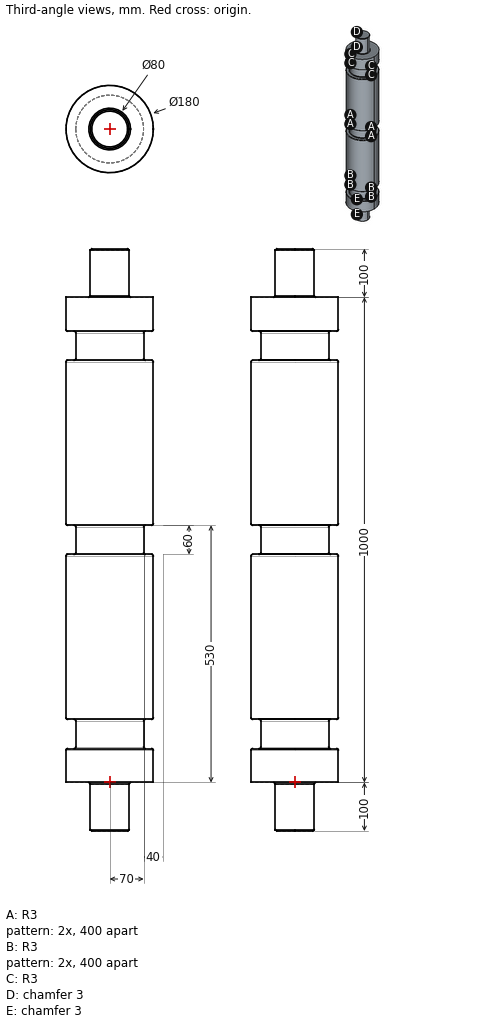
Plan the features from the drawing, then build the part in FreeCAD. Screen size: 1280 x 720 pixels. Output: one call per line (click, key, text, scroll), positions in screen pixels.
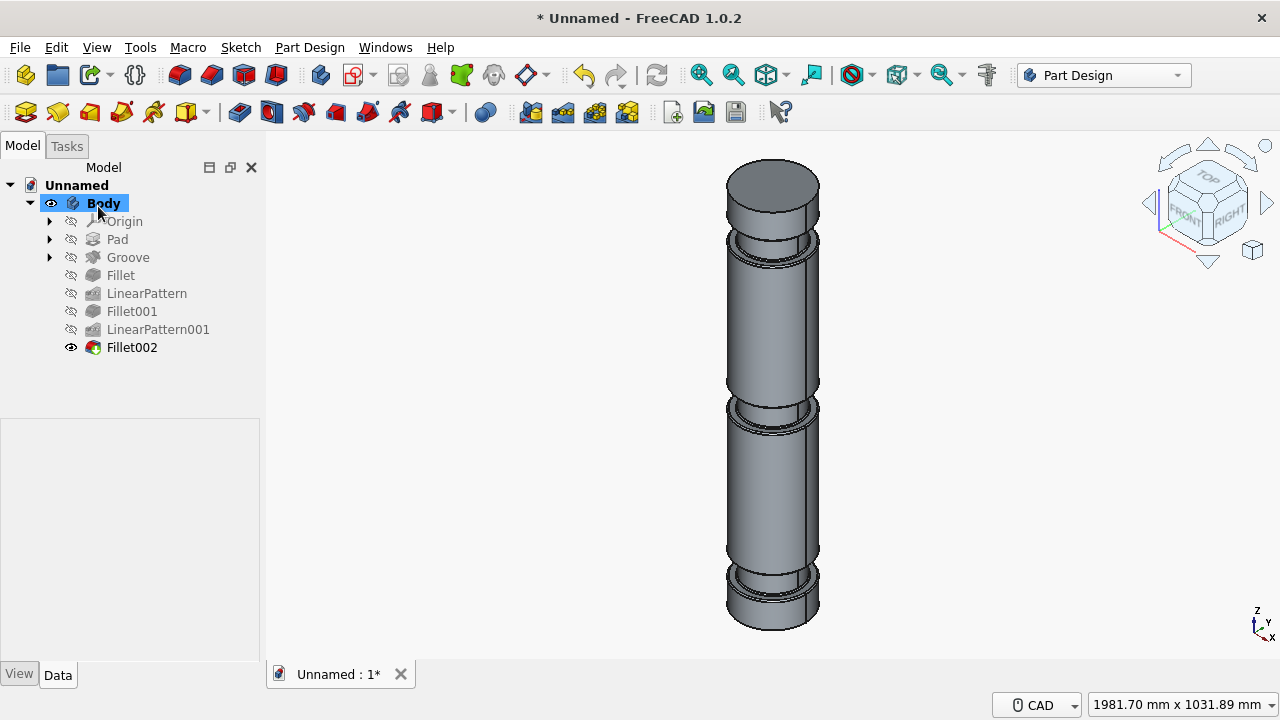
click(773, 185)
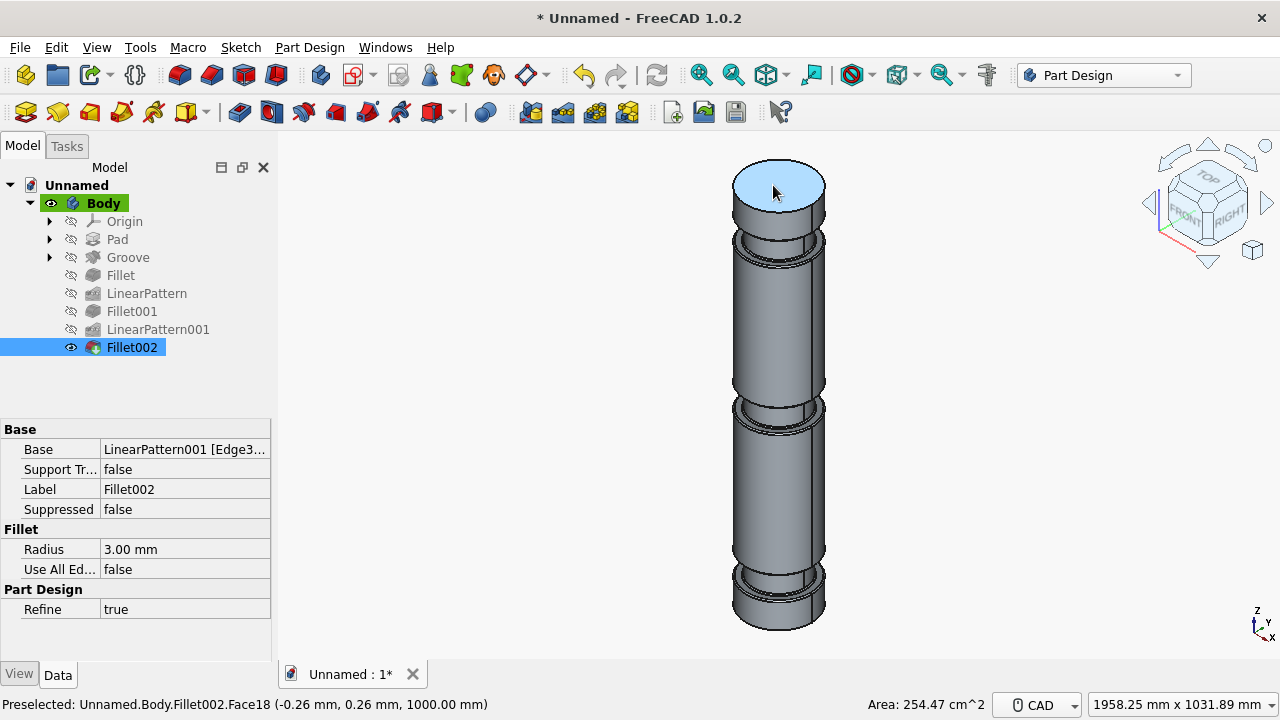
click(354, 76)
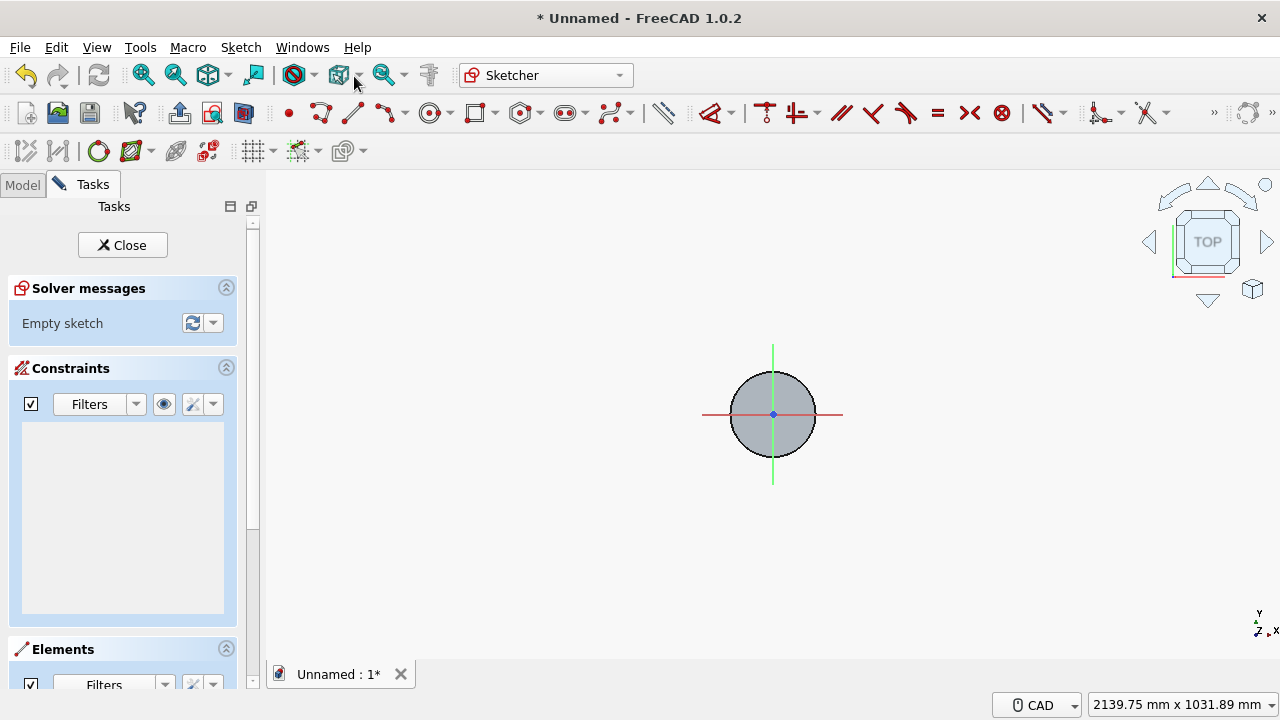
scroll(784, 415, up, 10)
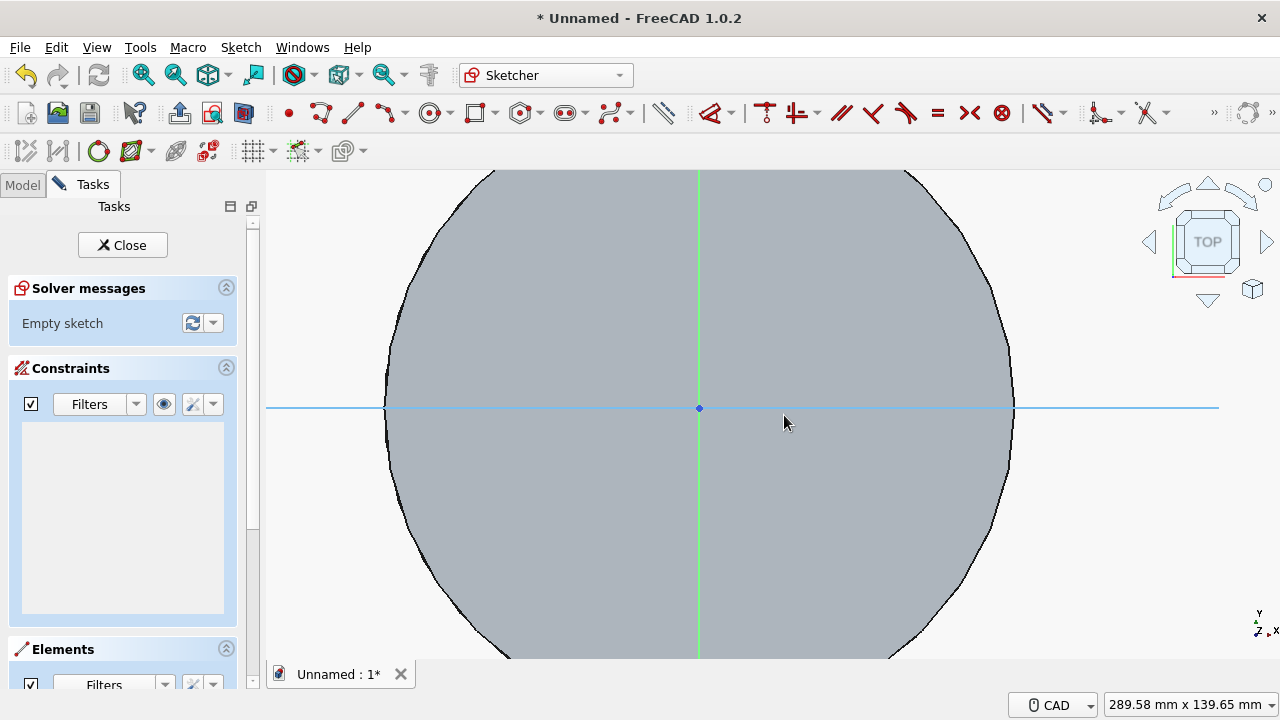
click(430, 114)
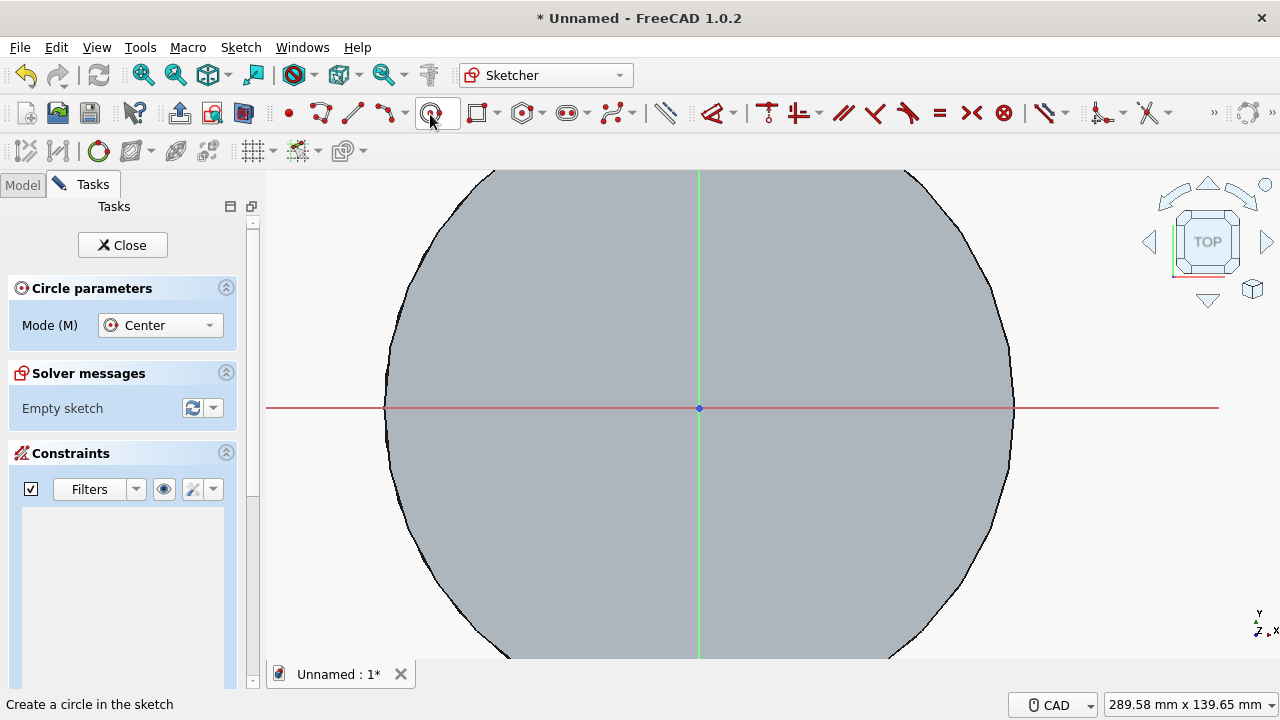
click(699, 408)
move(798, 309)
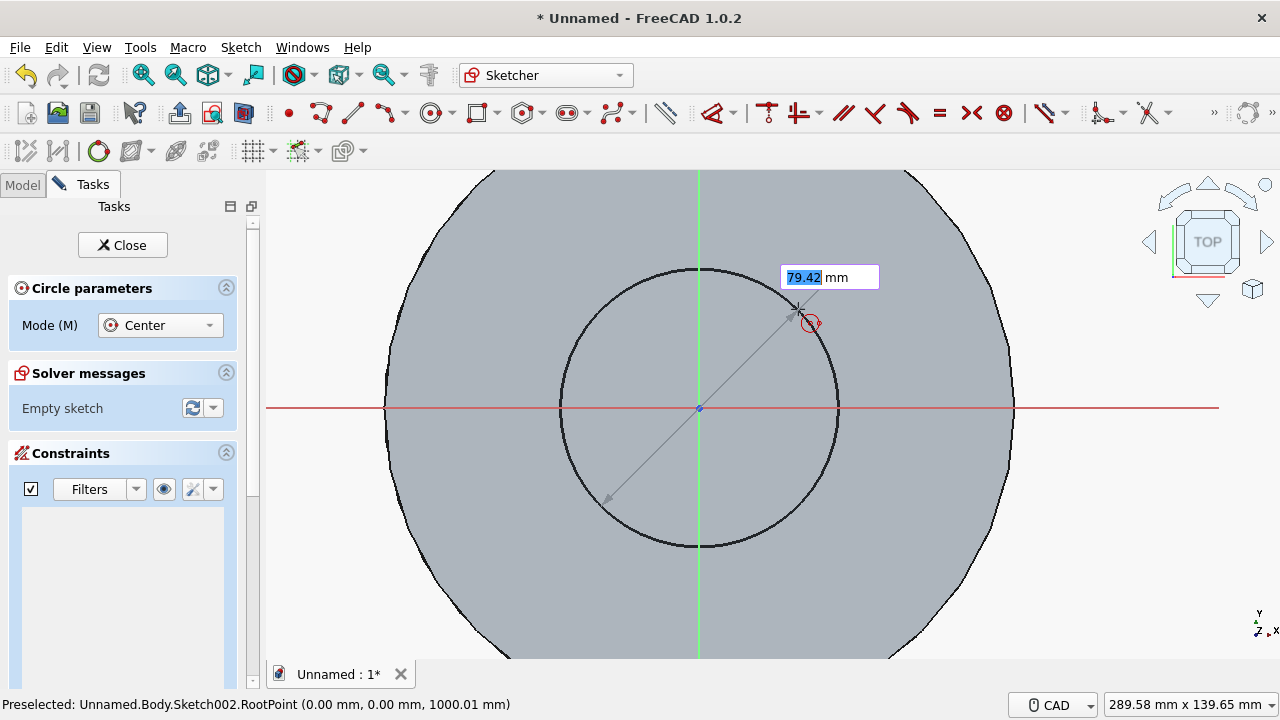
text(80)
key(Return)
key(Escape)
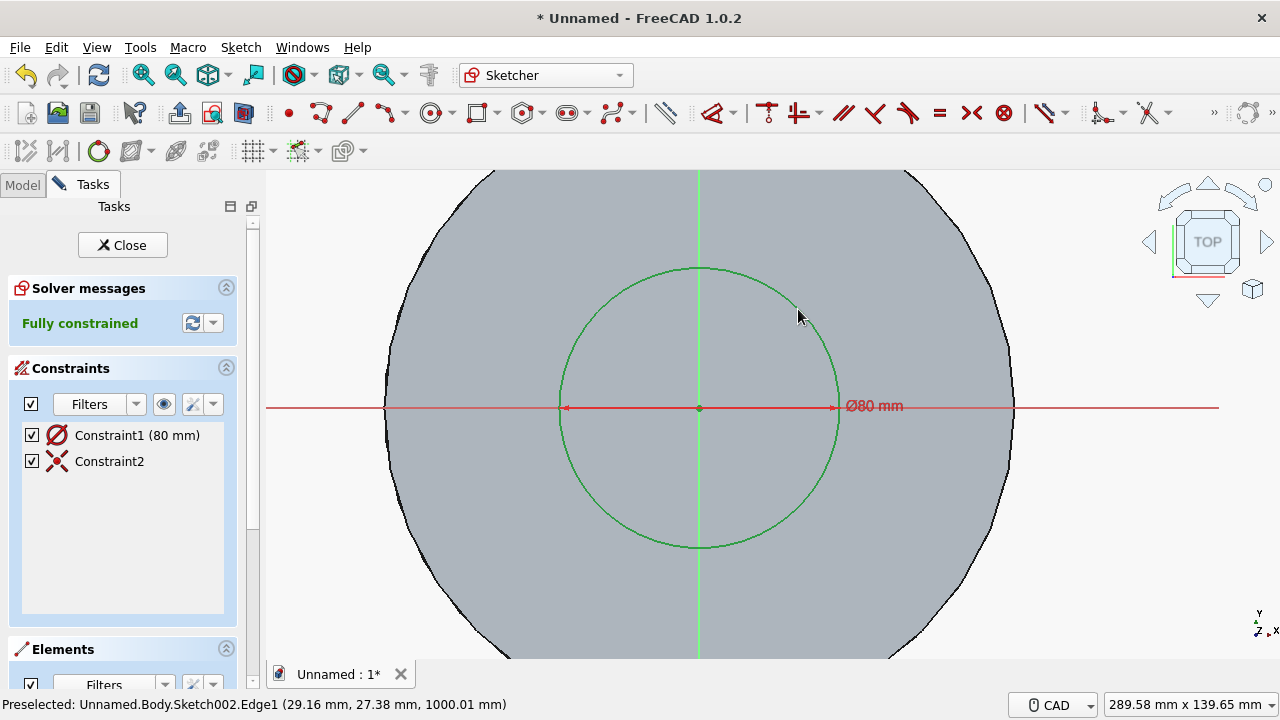
click(123, 245)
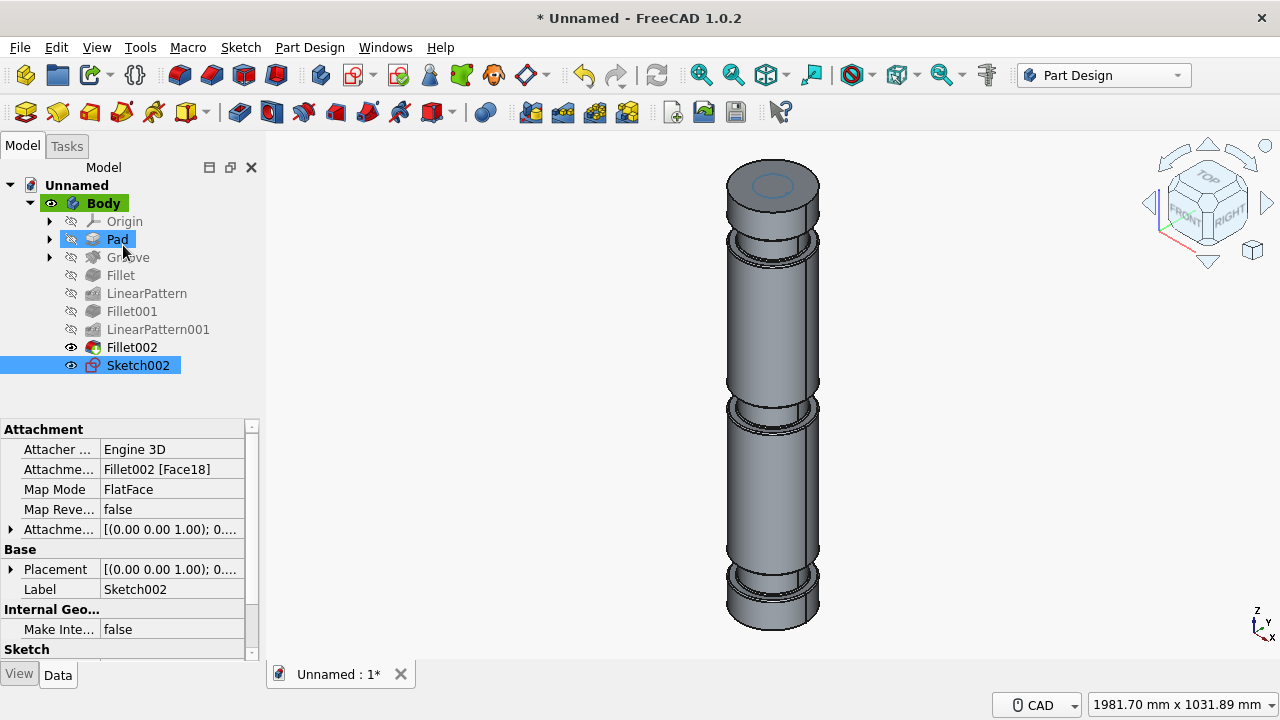
click(26, 112)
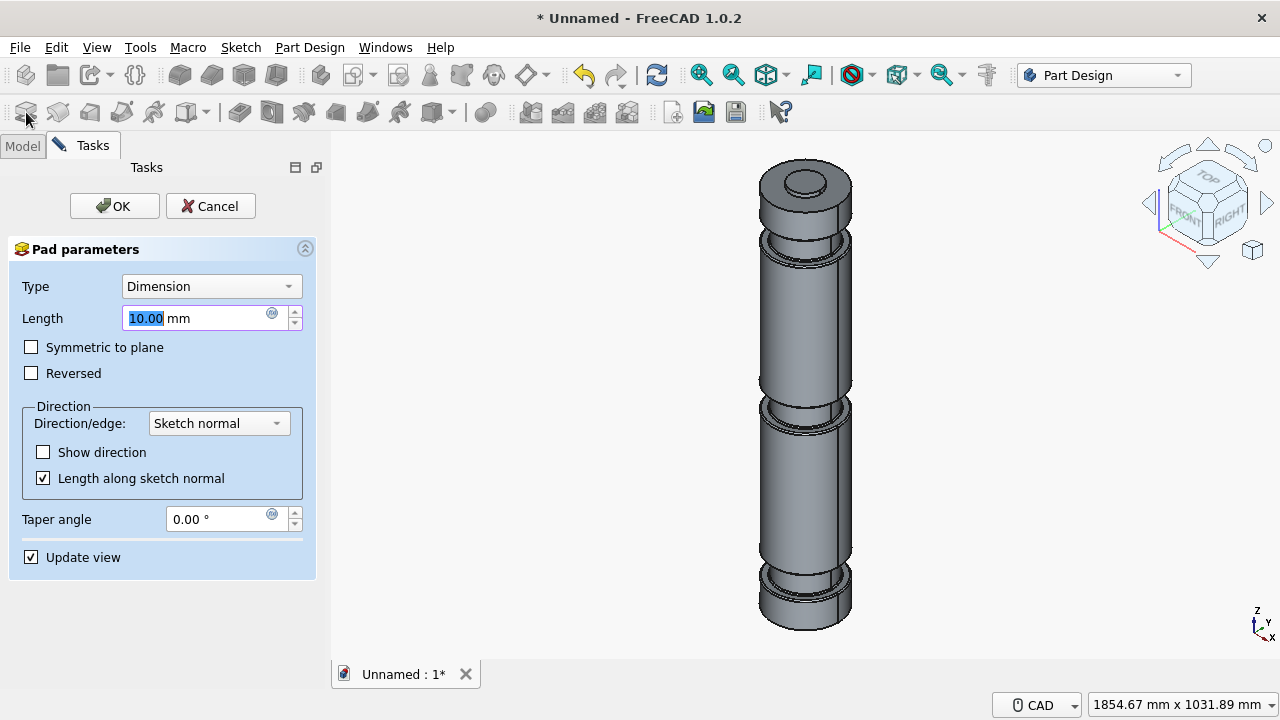
text(100)
key(Tab)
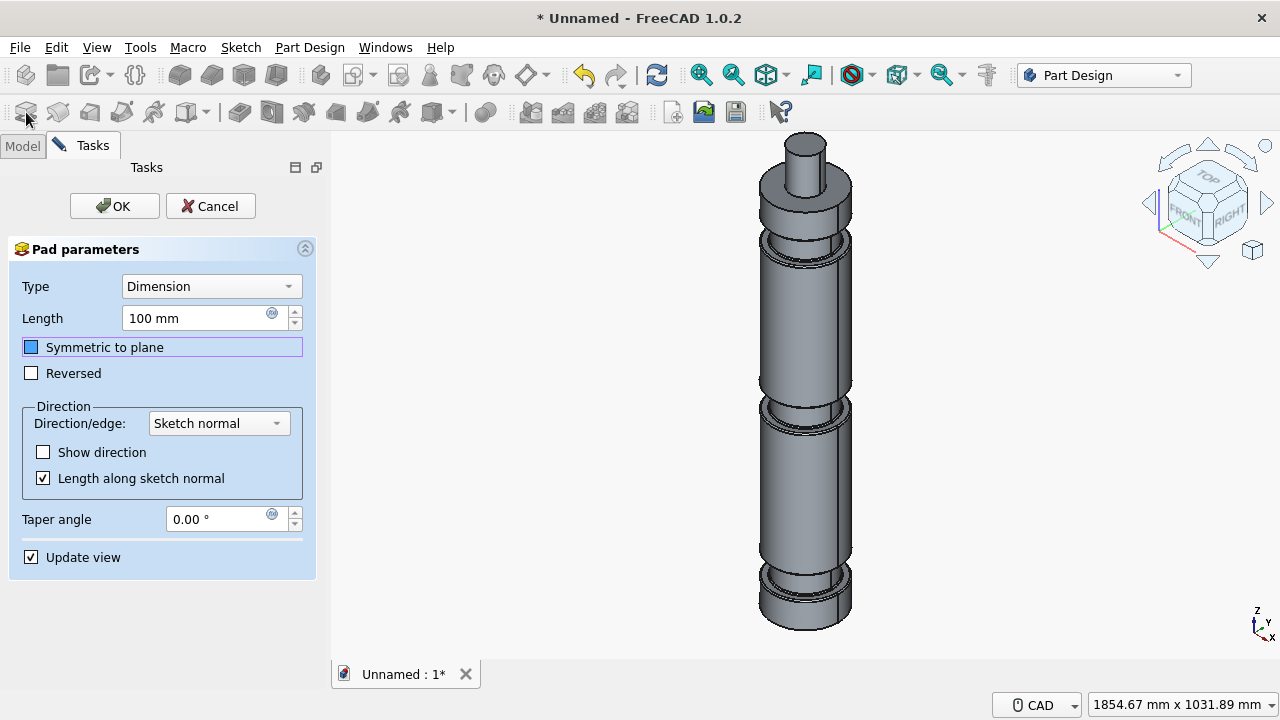
click(115, 206)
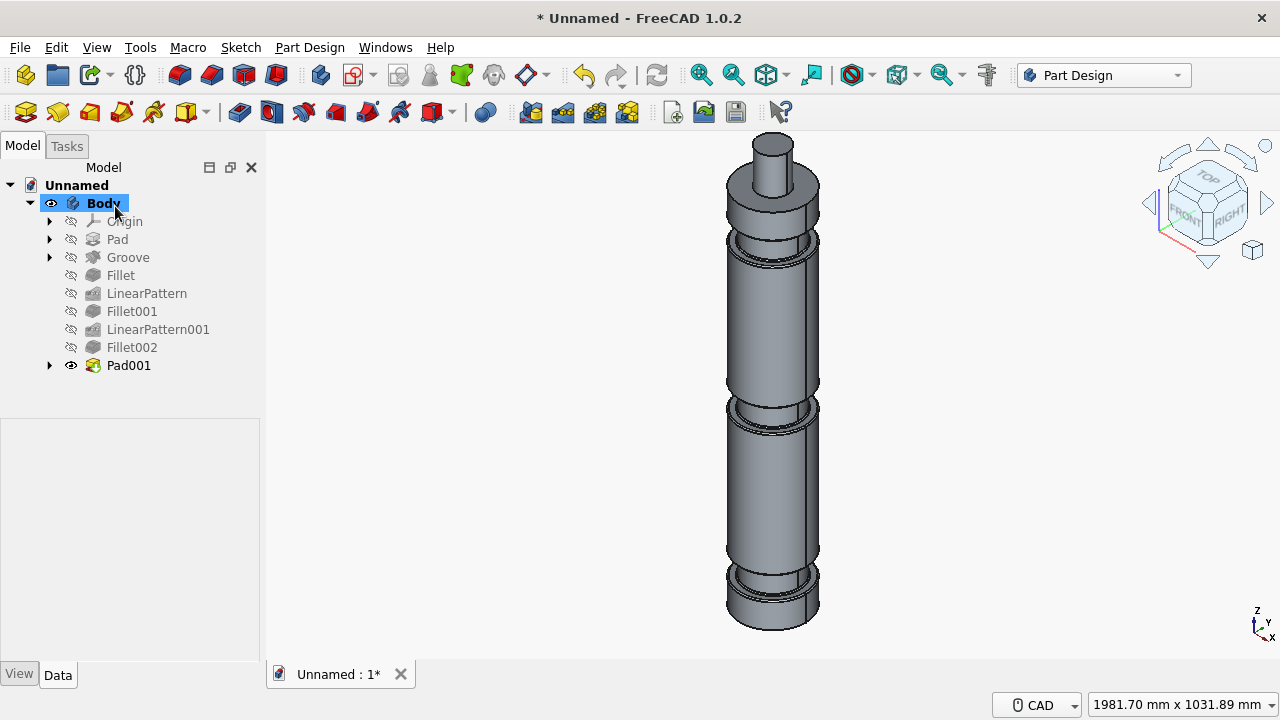
click(702, 76)